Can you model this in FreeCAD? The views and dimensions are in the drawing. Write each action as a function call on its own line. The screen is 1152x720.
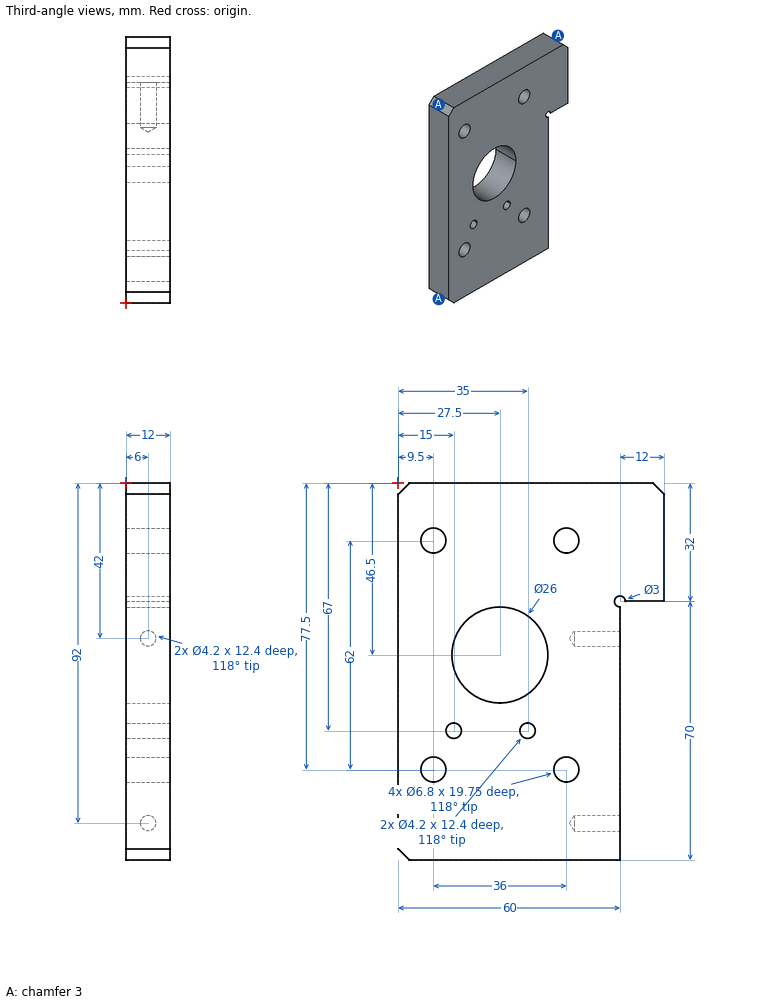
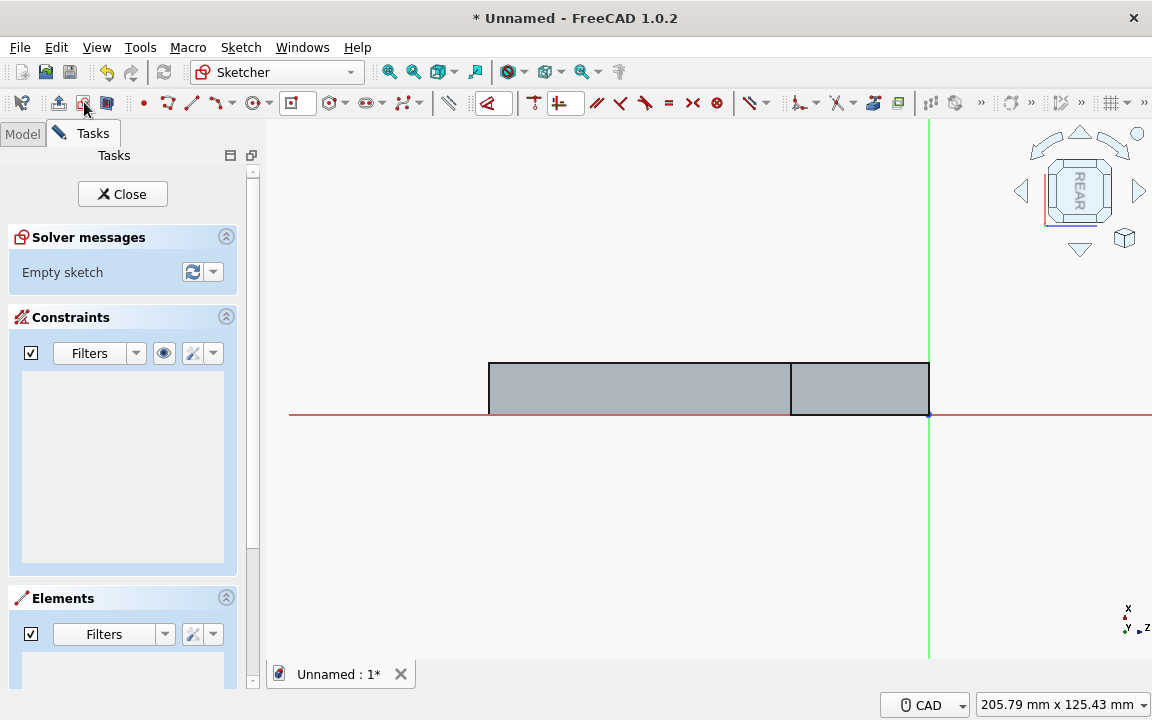
key(q)
key(s)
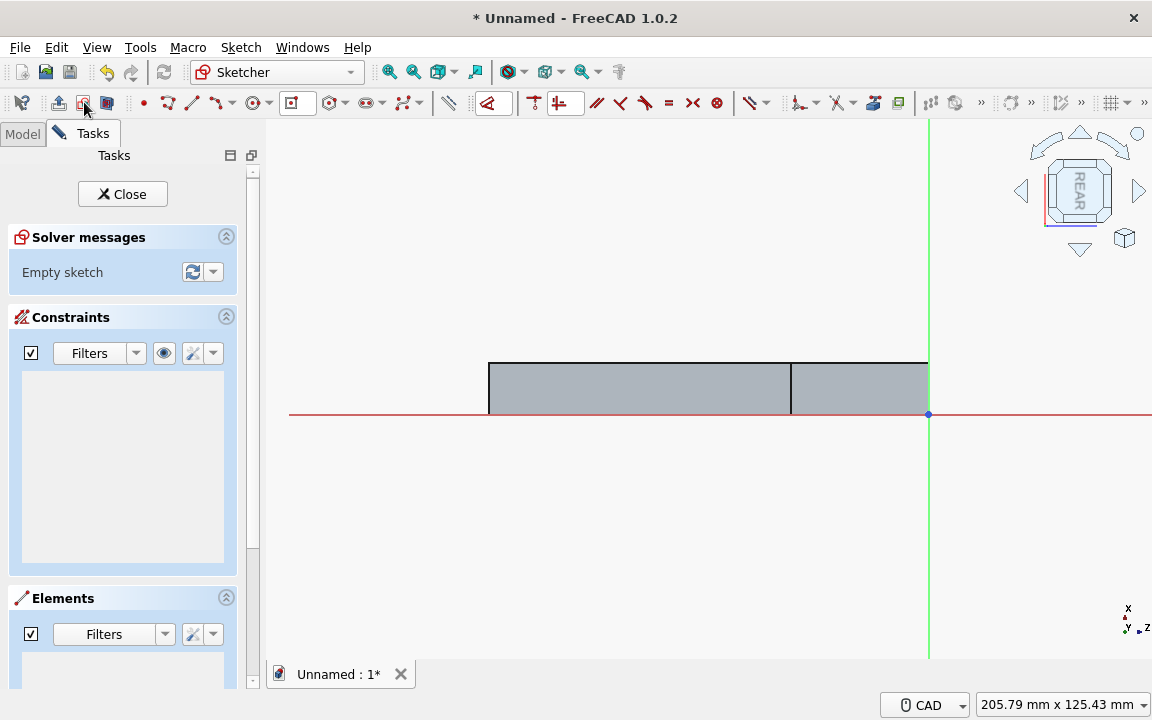
click(254, 104)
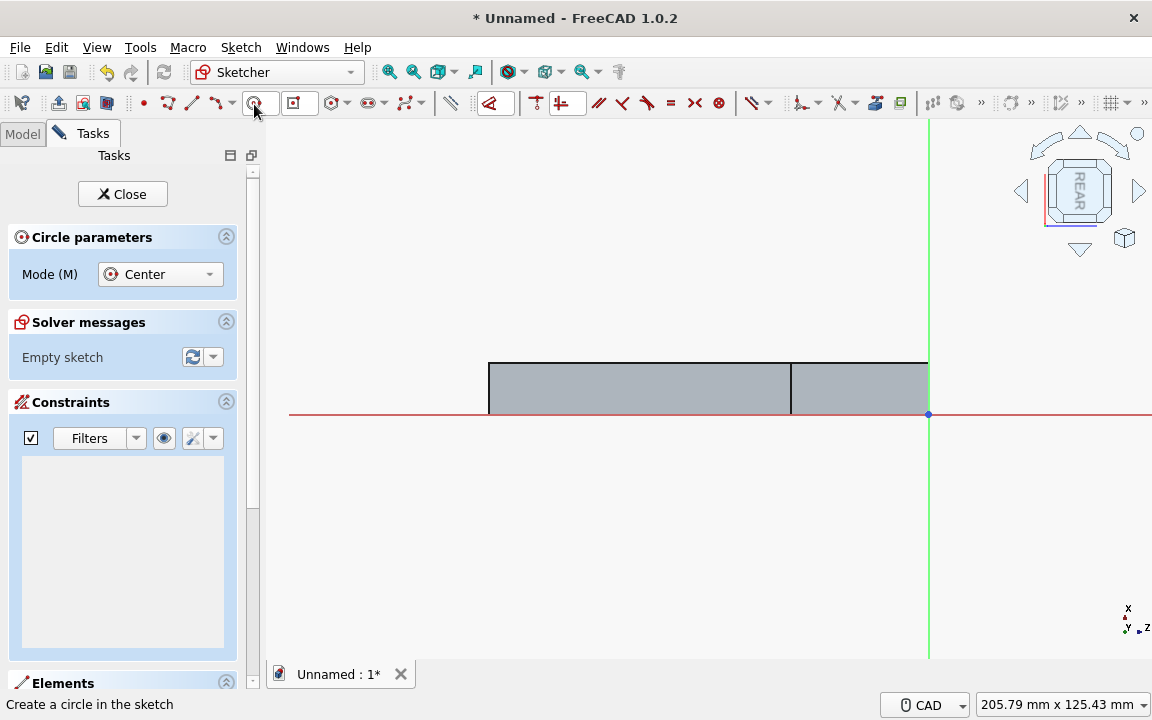
scroll(748, 389, up, 5)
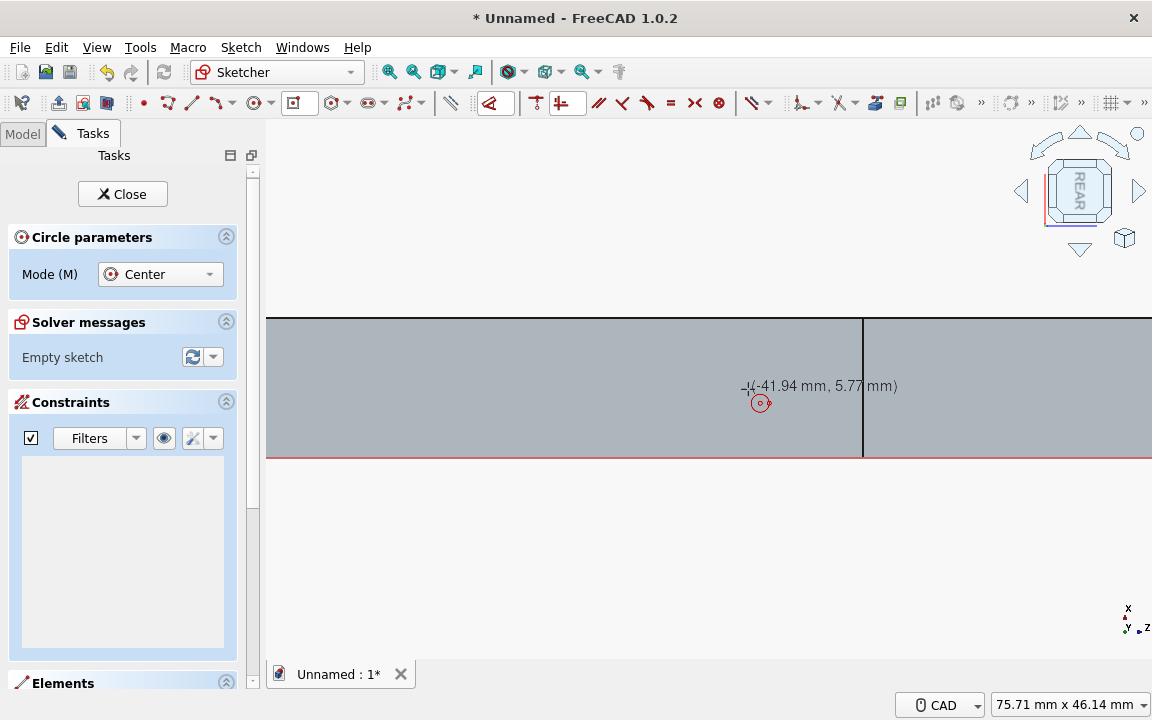
click(746, 388)
move(764, 371)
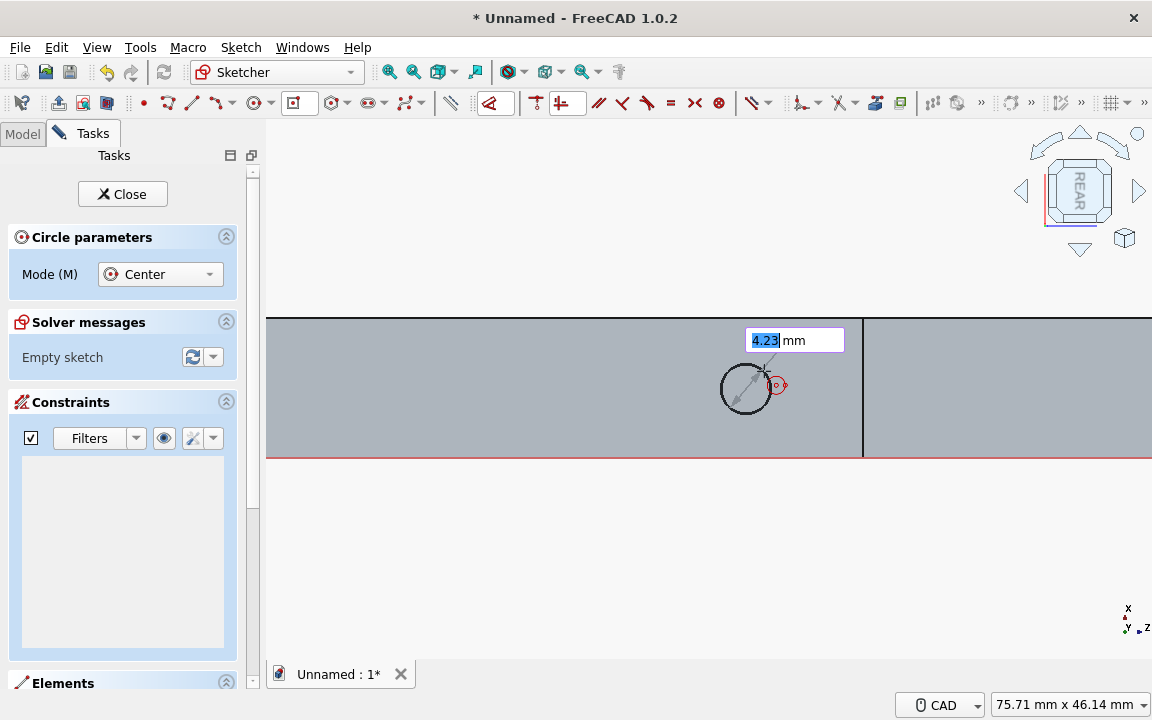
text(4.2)
key(Return)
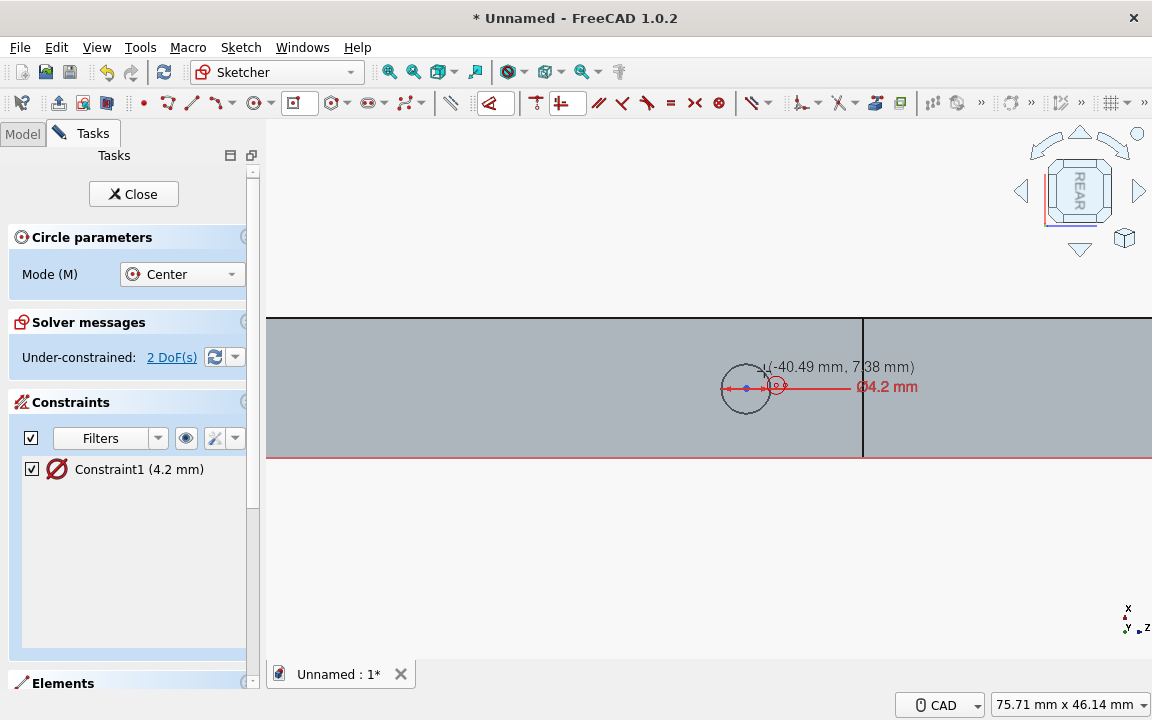
scroll(602, 371, down, 4)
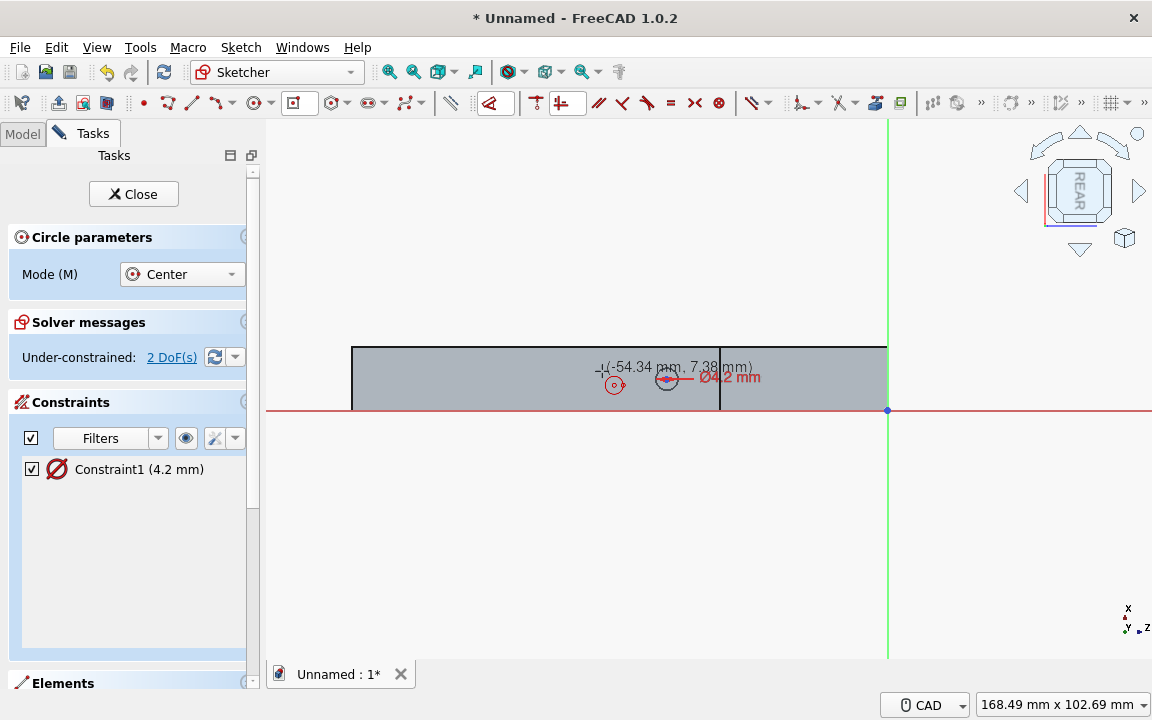
scroll(404, 379, up, 4)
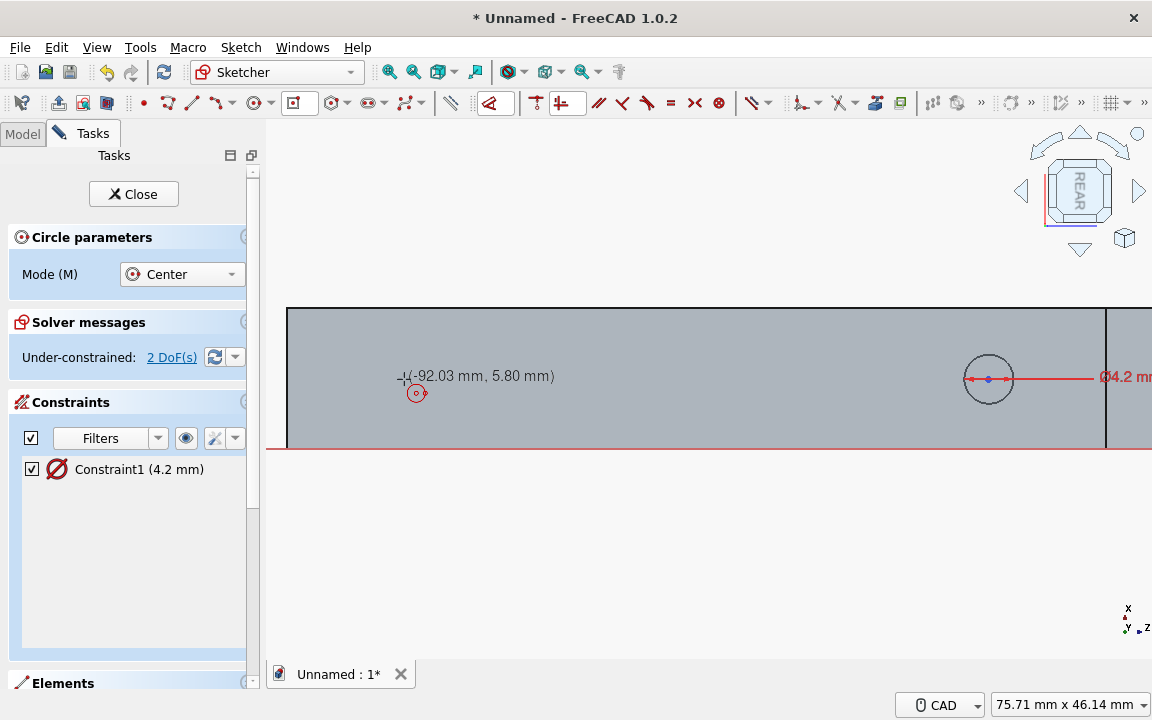
click(404, 378)
move(422, 361)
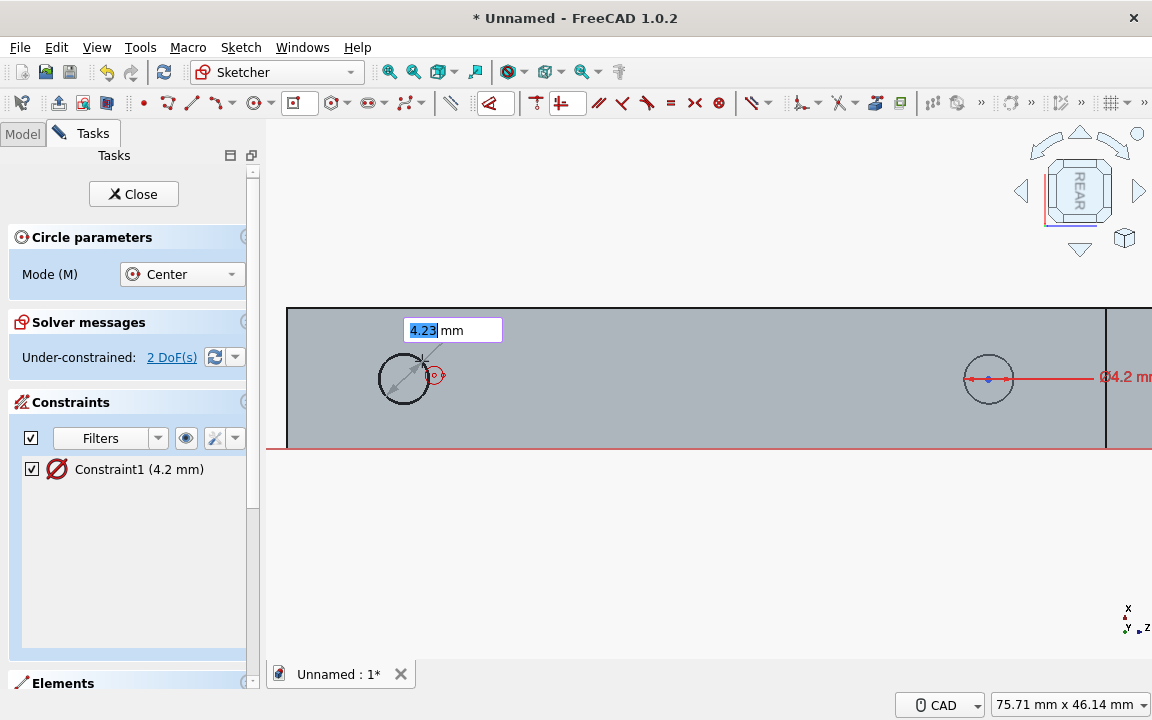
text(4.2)
key(Return)
key(Escape)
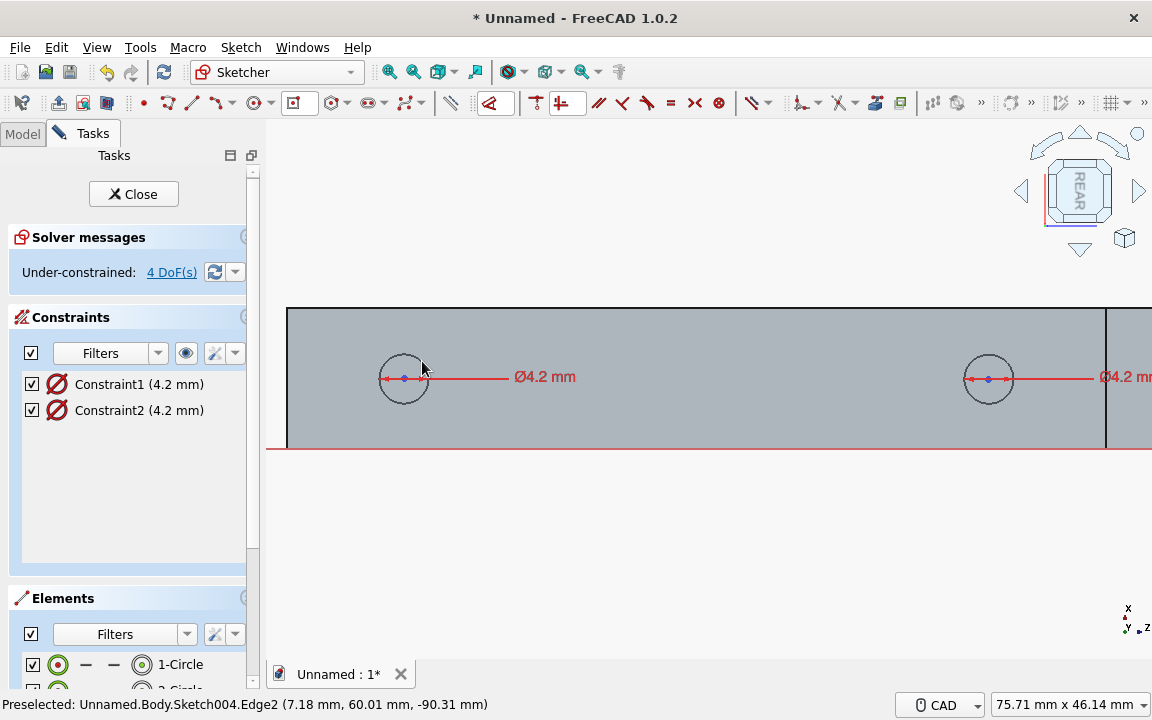
scroll(404, 379, down, 4)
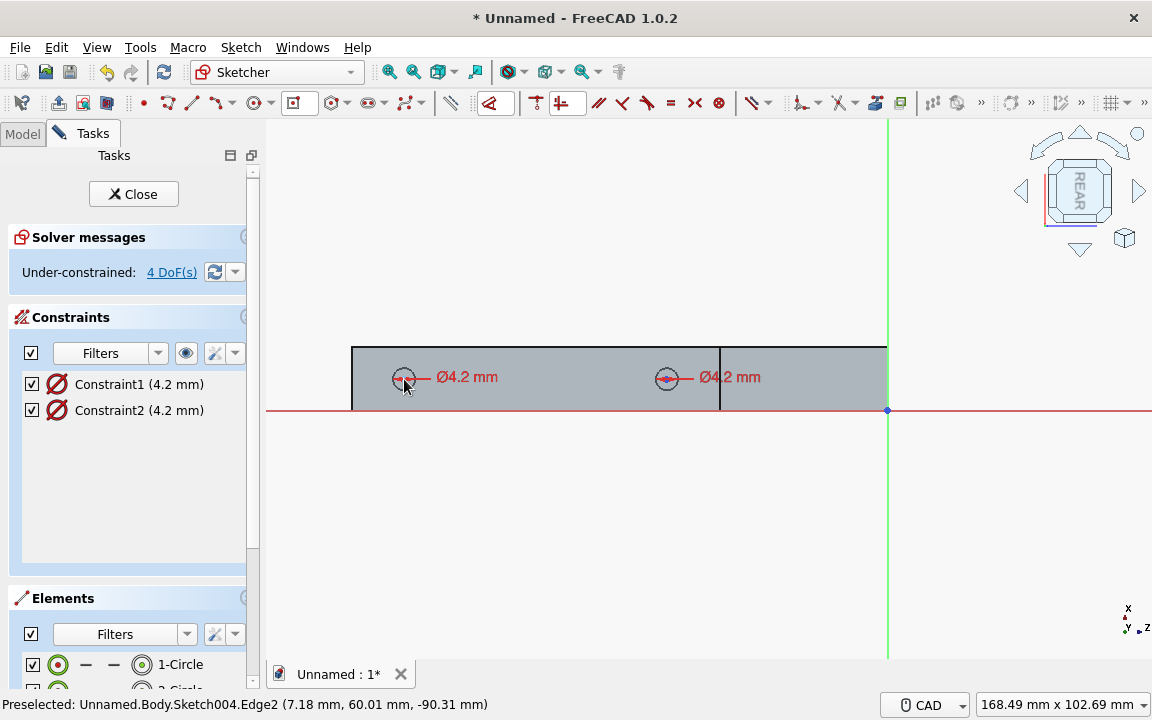
click(667, 379)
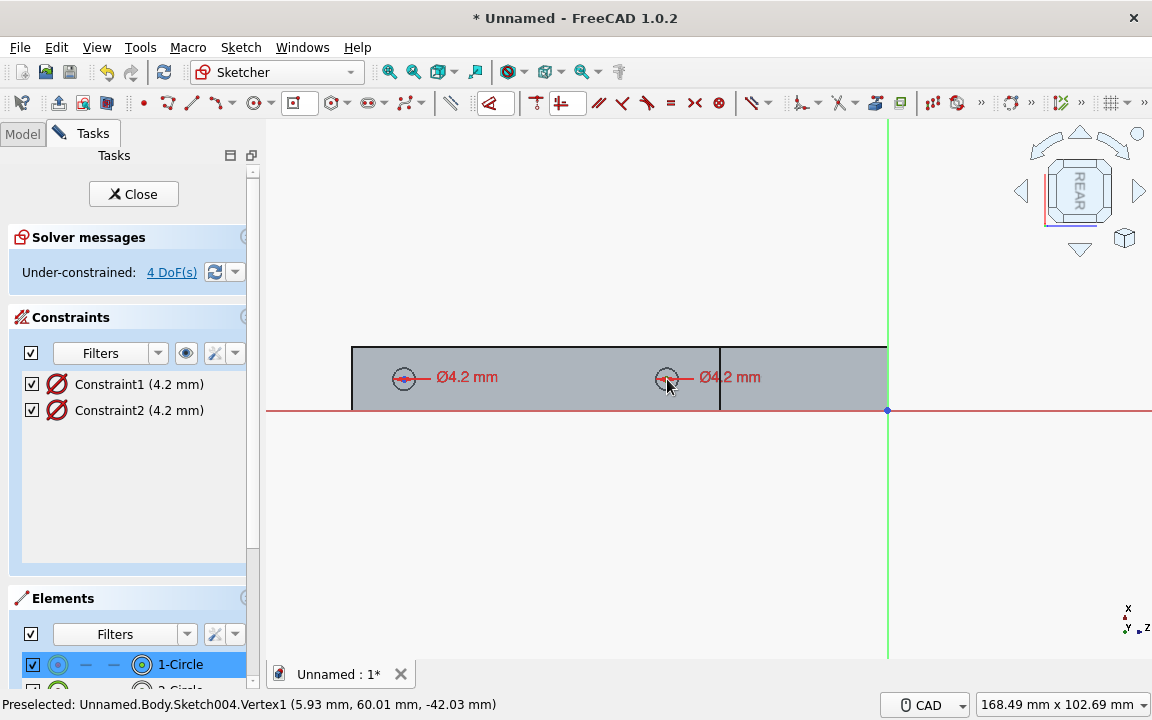
click(404, 379)